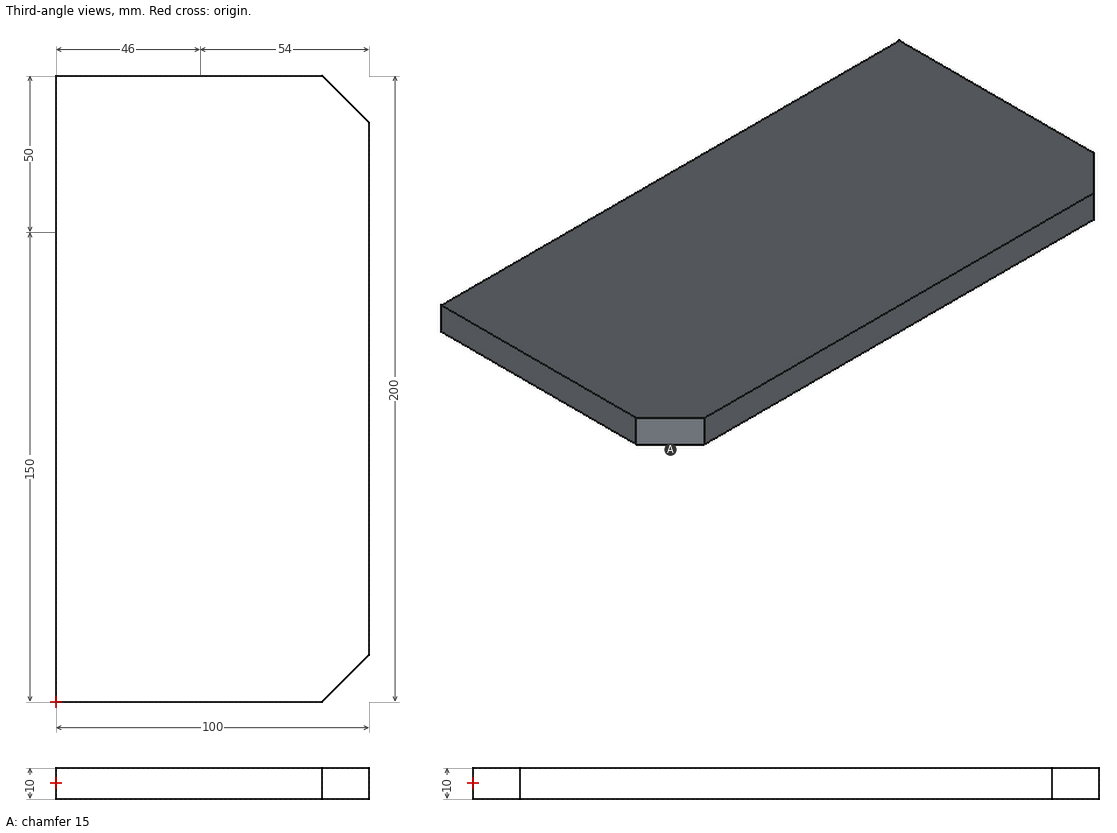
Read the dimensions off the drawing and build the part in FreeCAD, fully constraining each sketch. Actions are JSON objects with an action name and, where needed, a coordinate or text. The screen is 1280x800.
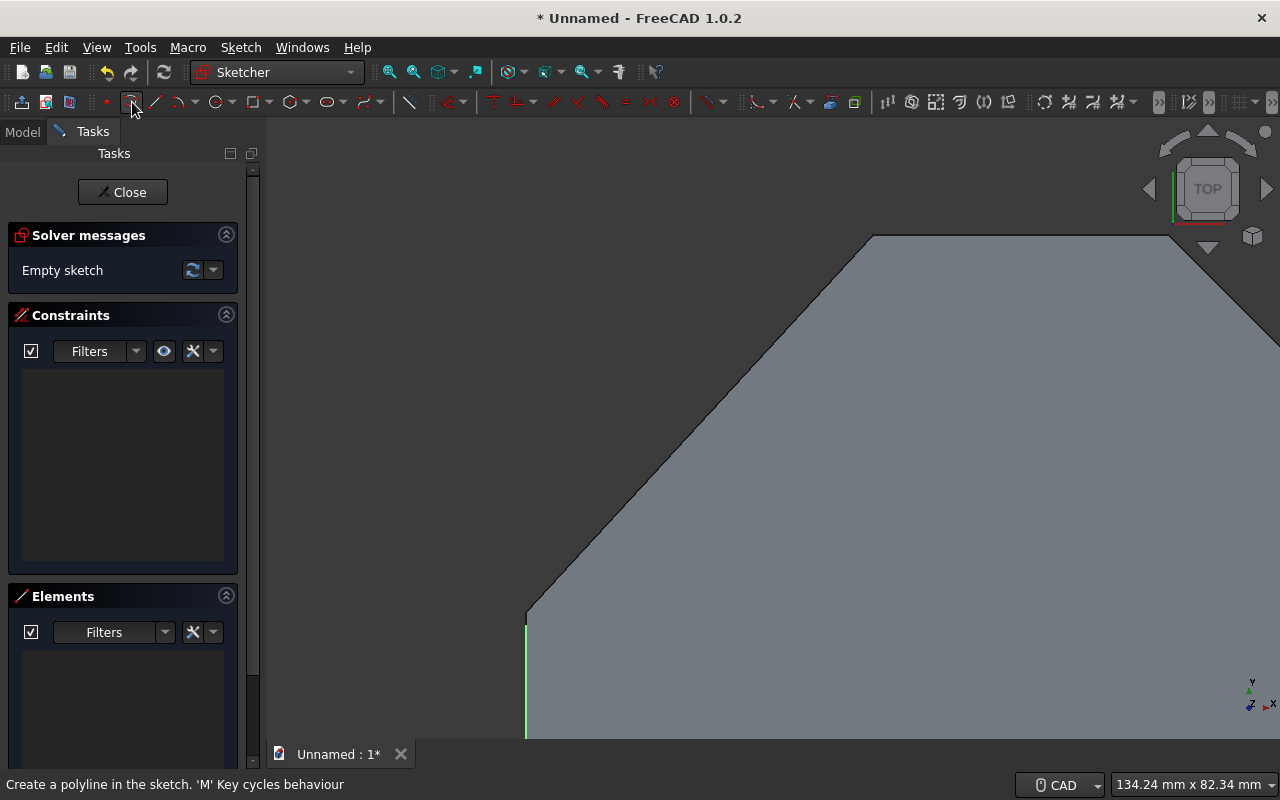
{"action": "left_click", "coordinate": [526, 613]}
{"action": "left_click", "coordinate": [873, 235]}
{"action": "left_click", "coordinate": [535, 235]}
{"action": "left_click", "coordinate": [526, 614]}
{"action": "key", "text": "Escape"}
{"action": "key", "text": "Escape"}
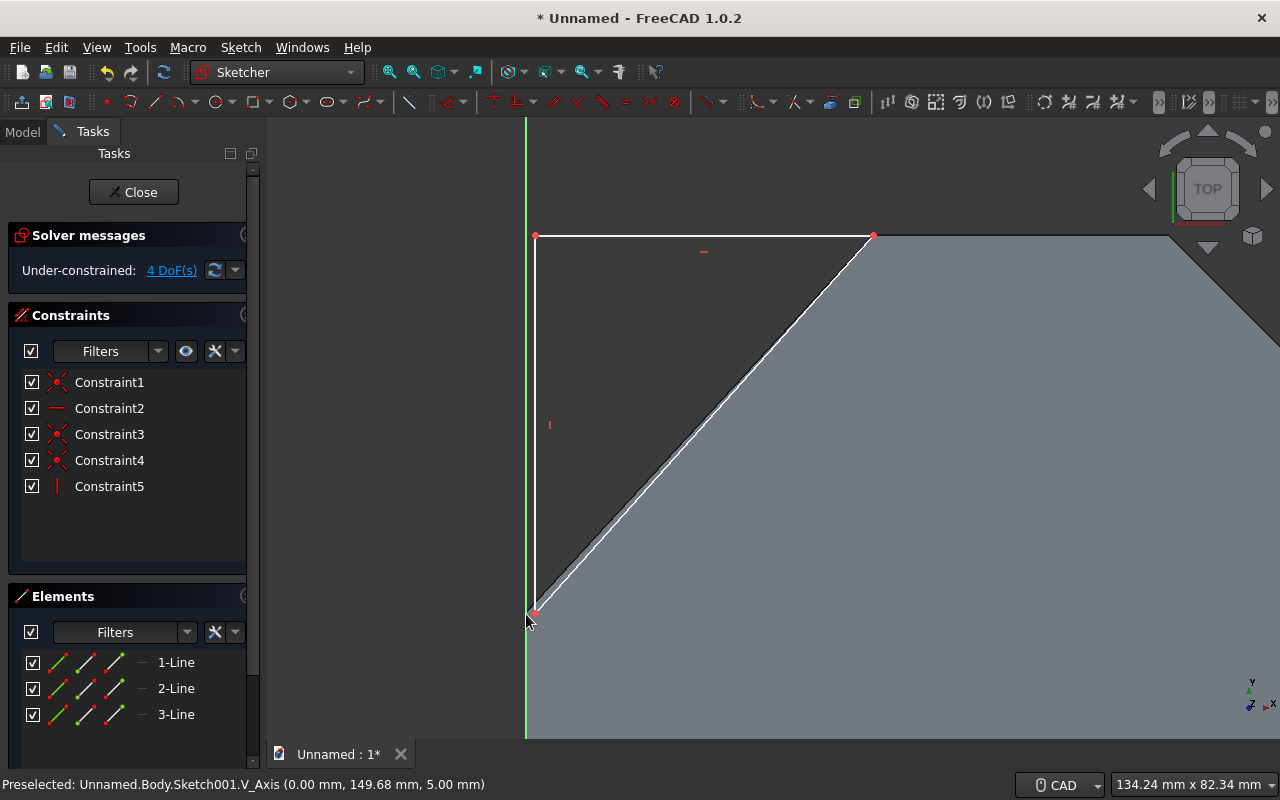
{"action": "left_click", "coordinate": [535, 614]}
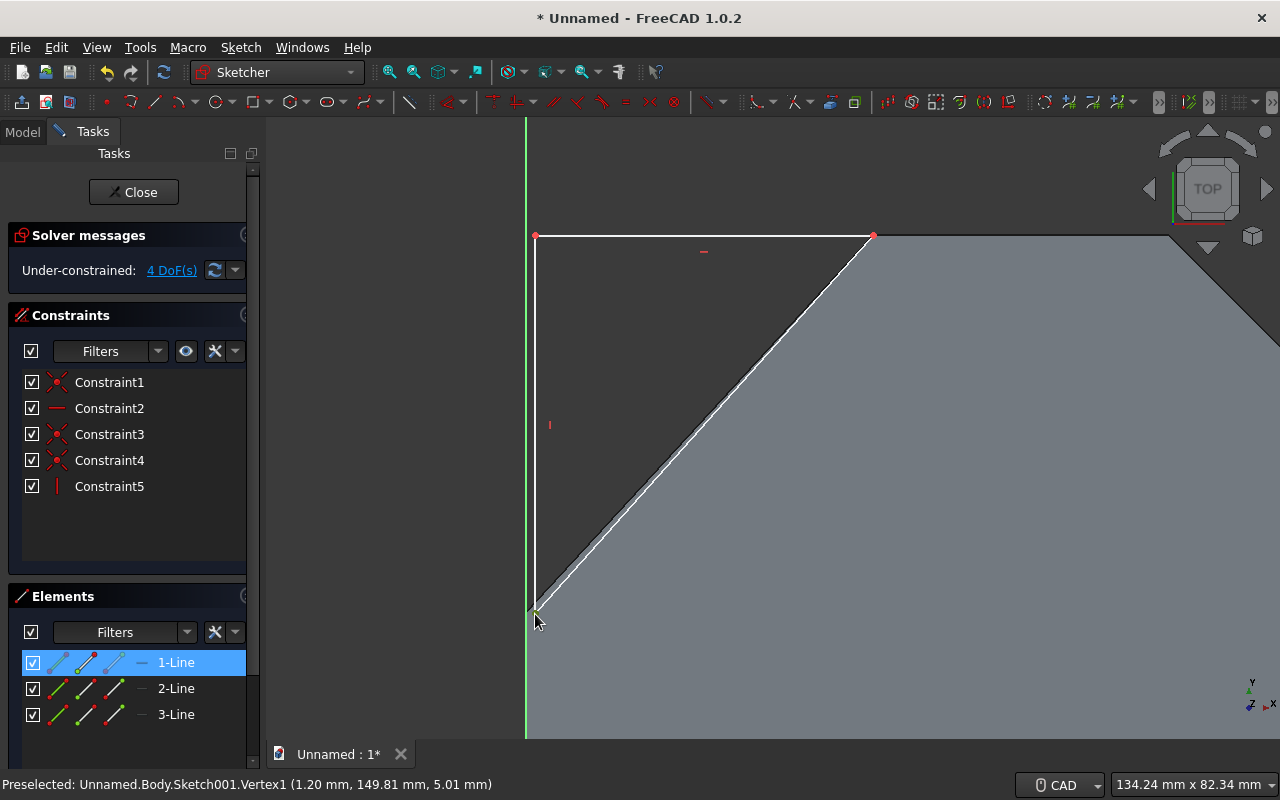
{"action": "left_click", "coordinate": [526, 671]}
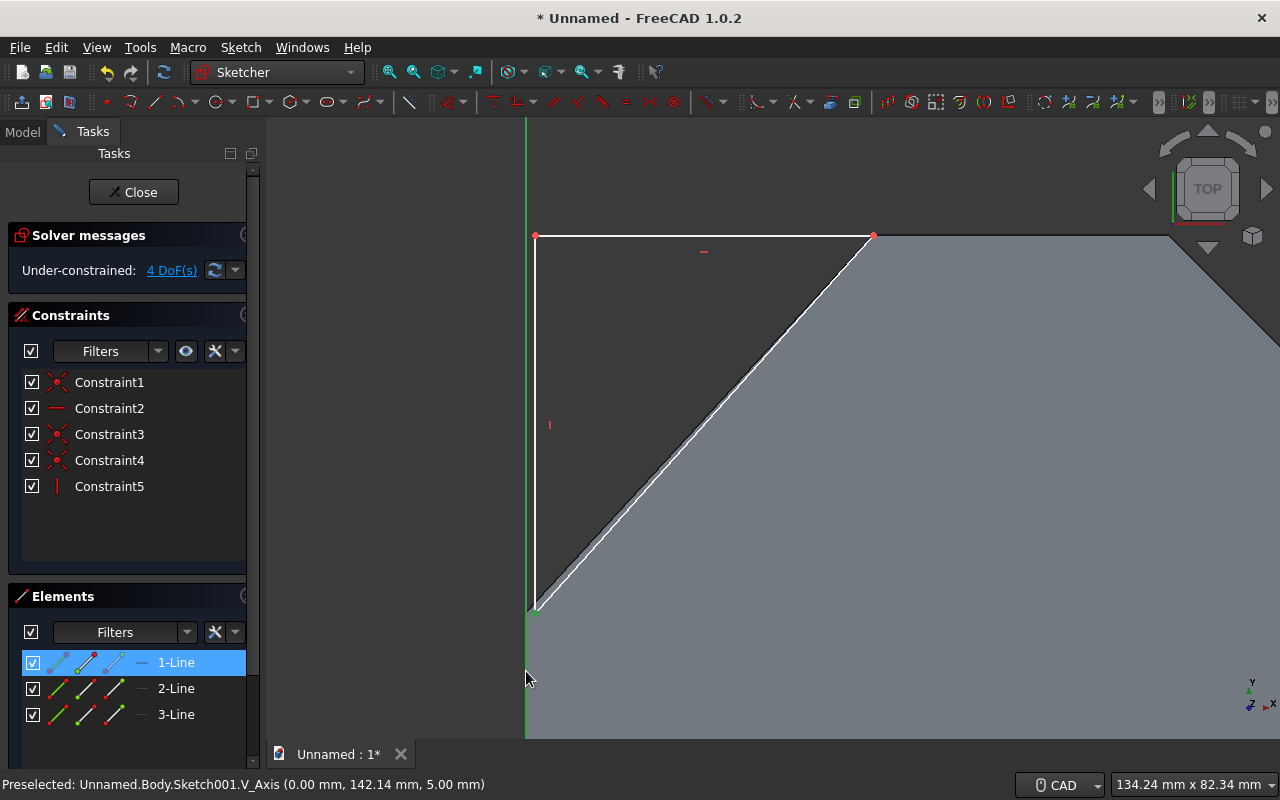
{"action": "left_click", "coordinate": [494, 102]}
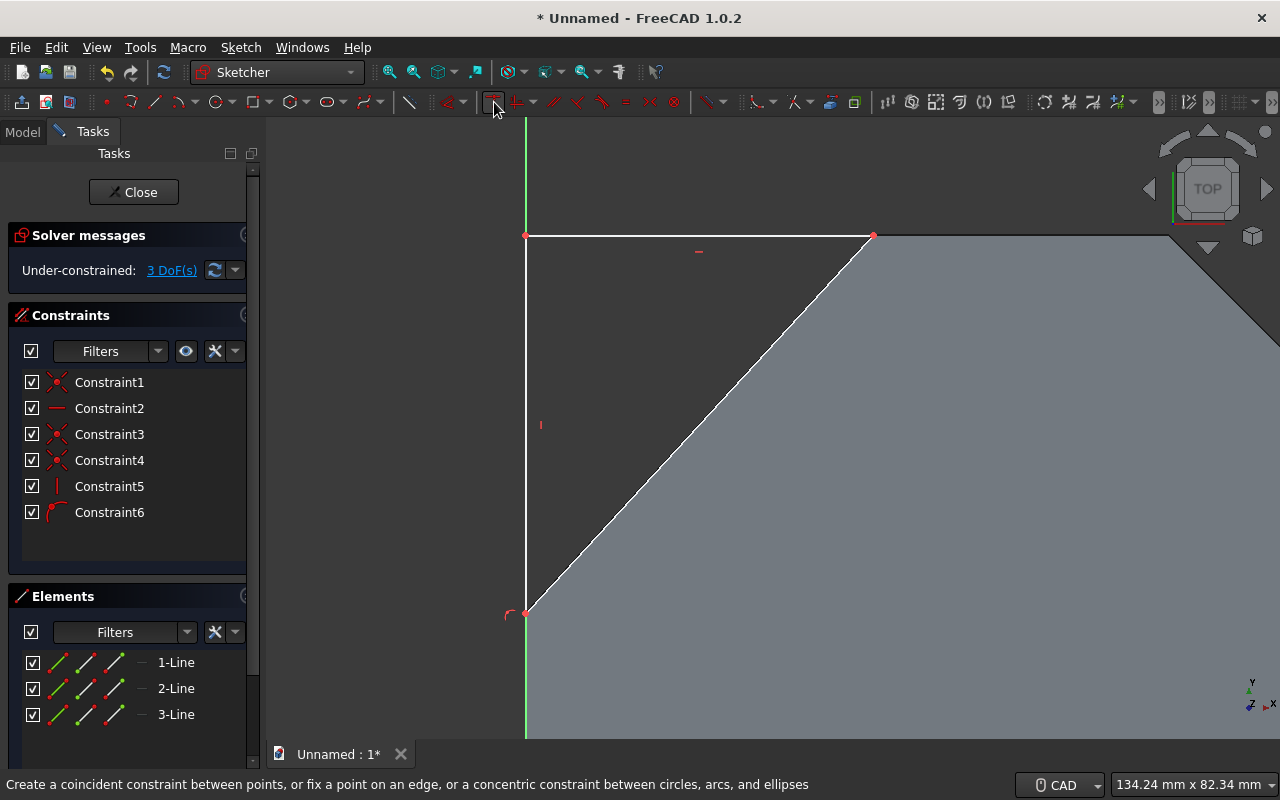
{"action": "left_click", "coordinate": [448, 102]}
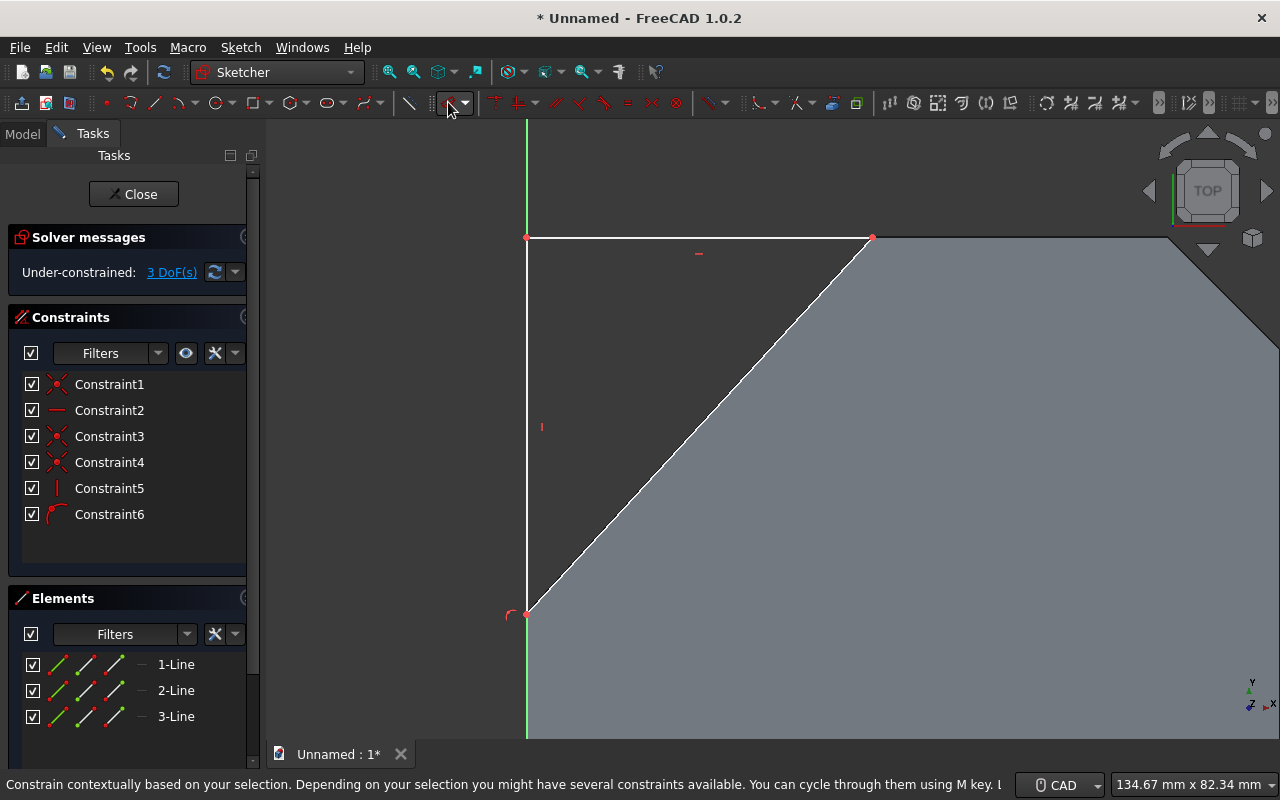
{"action": "left_click", "coordinate": [769, 238]}
{"action": "left_click", "coordinate": [700, 204]}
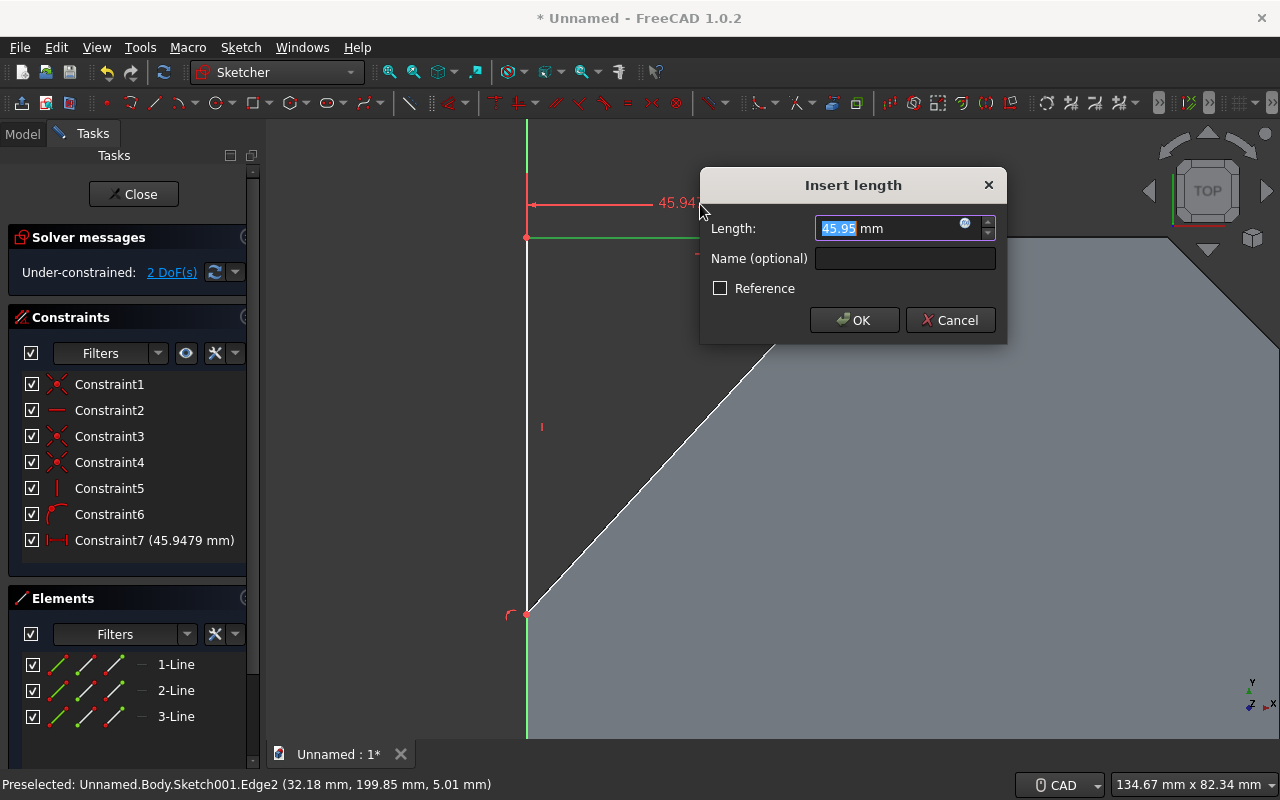
{"action": "type", "text": "46"}
{"action": "key", "text": "Return"}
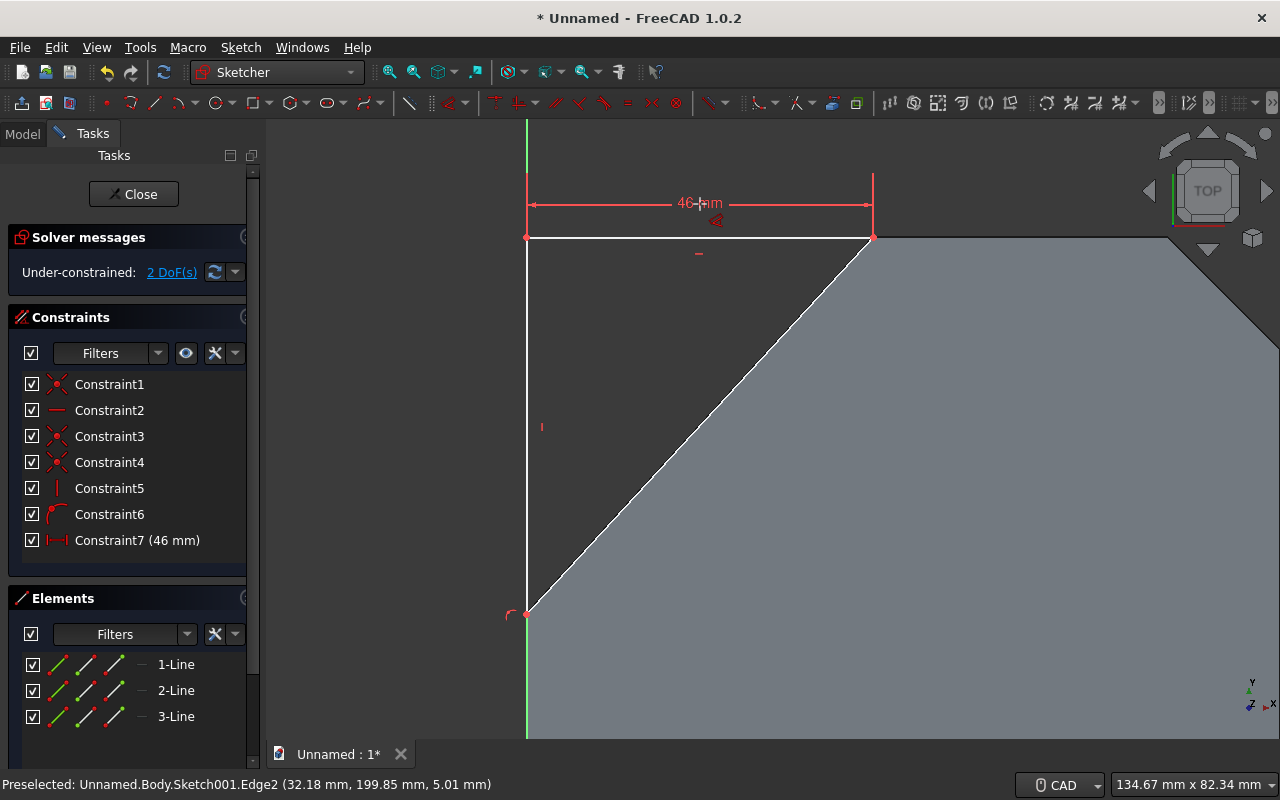
{"action": "left_click", "coordinate": [527, 351]}
{"action": "left_click", "coordinate": [493, 426]}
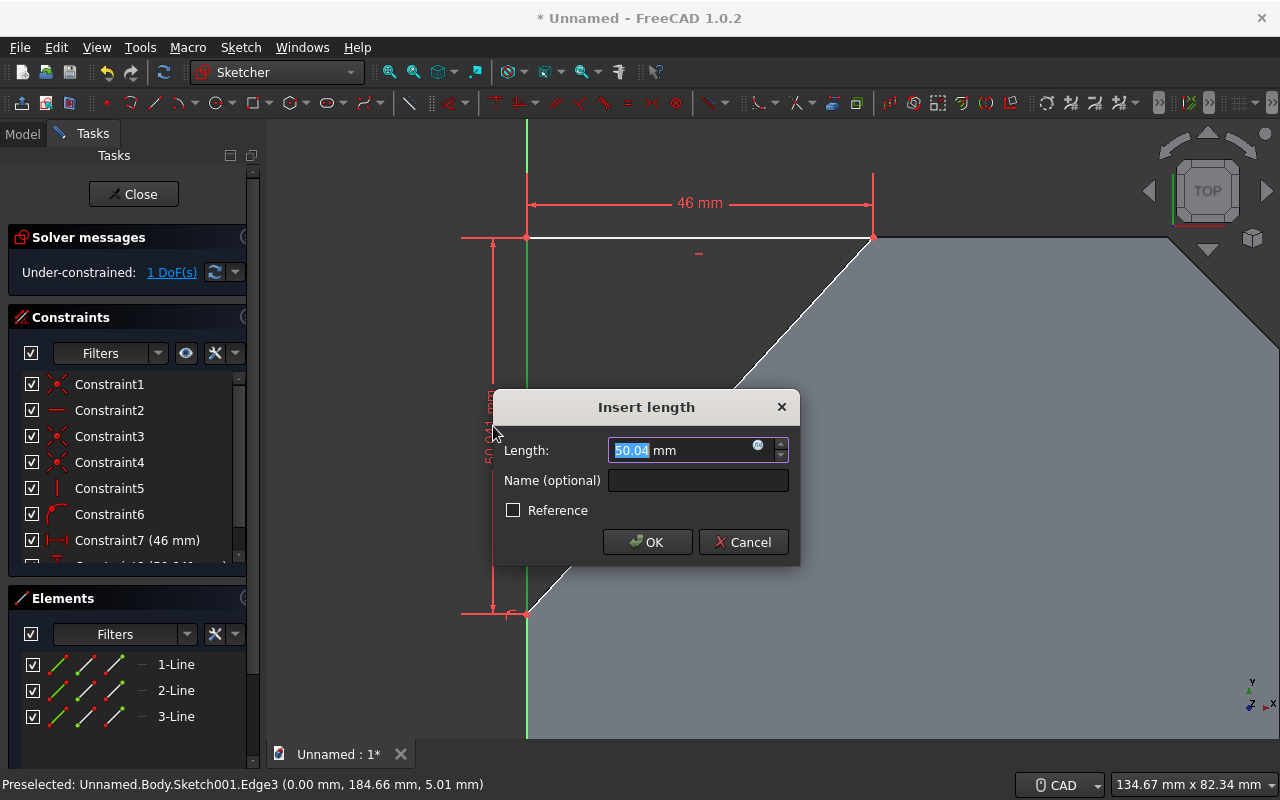
{"action": "type", "text": "50"}
{"action": "key", "text": "Return"}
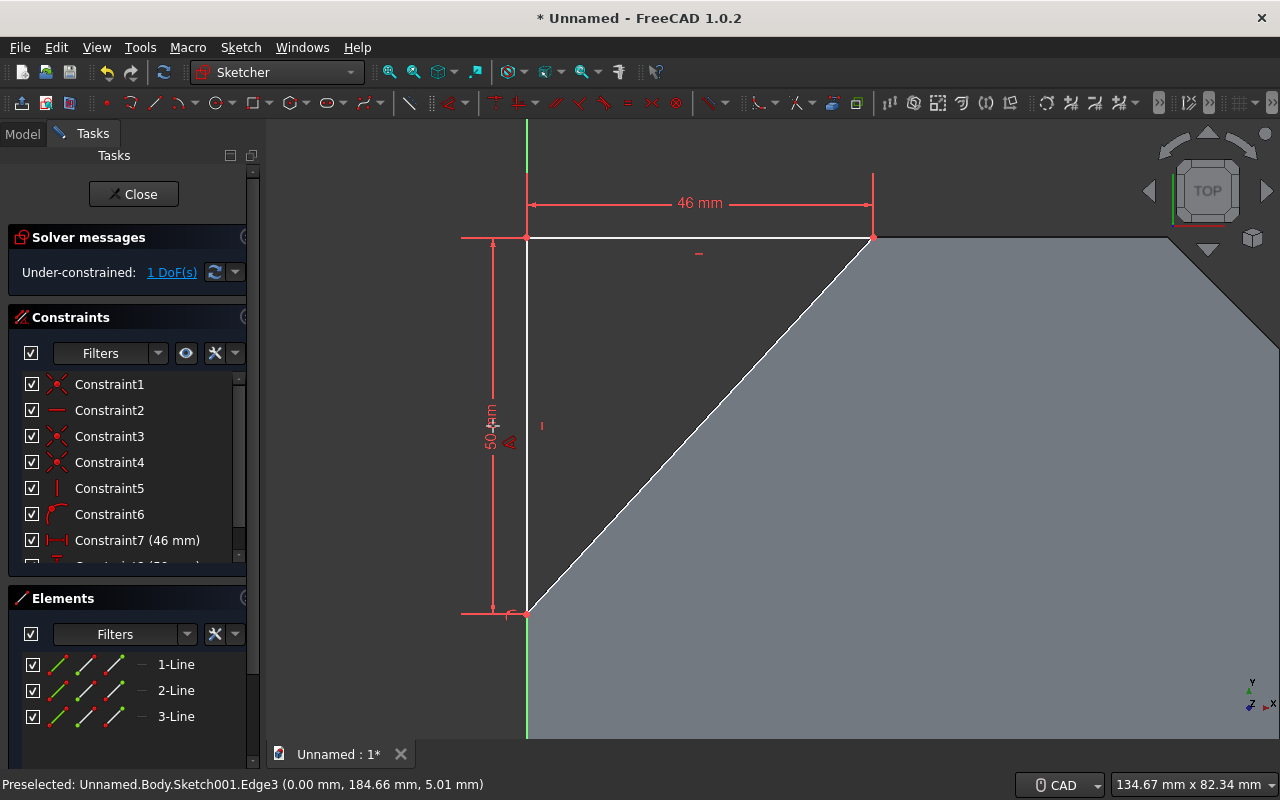
{"action": "left_click", "coordinate": [527, 614]}
{"action": "left_click", "coordinate": [493, 663]}